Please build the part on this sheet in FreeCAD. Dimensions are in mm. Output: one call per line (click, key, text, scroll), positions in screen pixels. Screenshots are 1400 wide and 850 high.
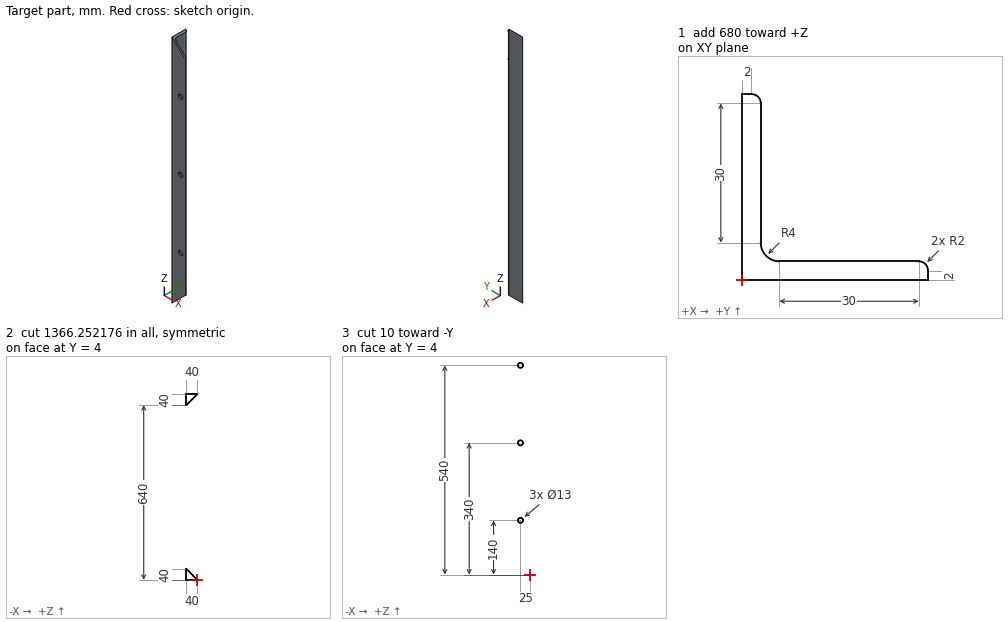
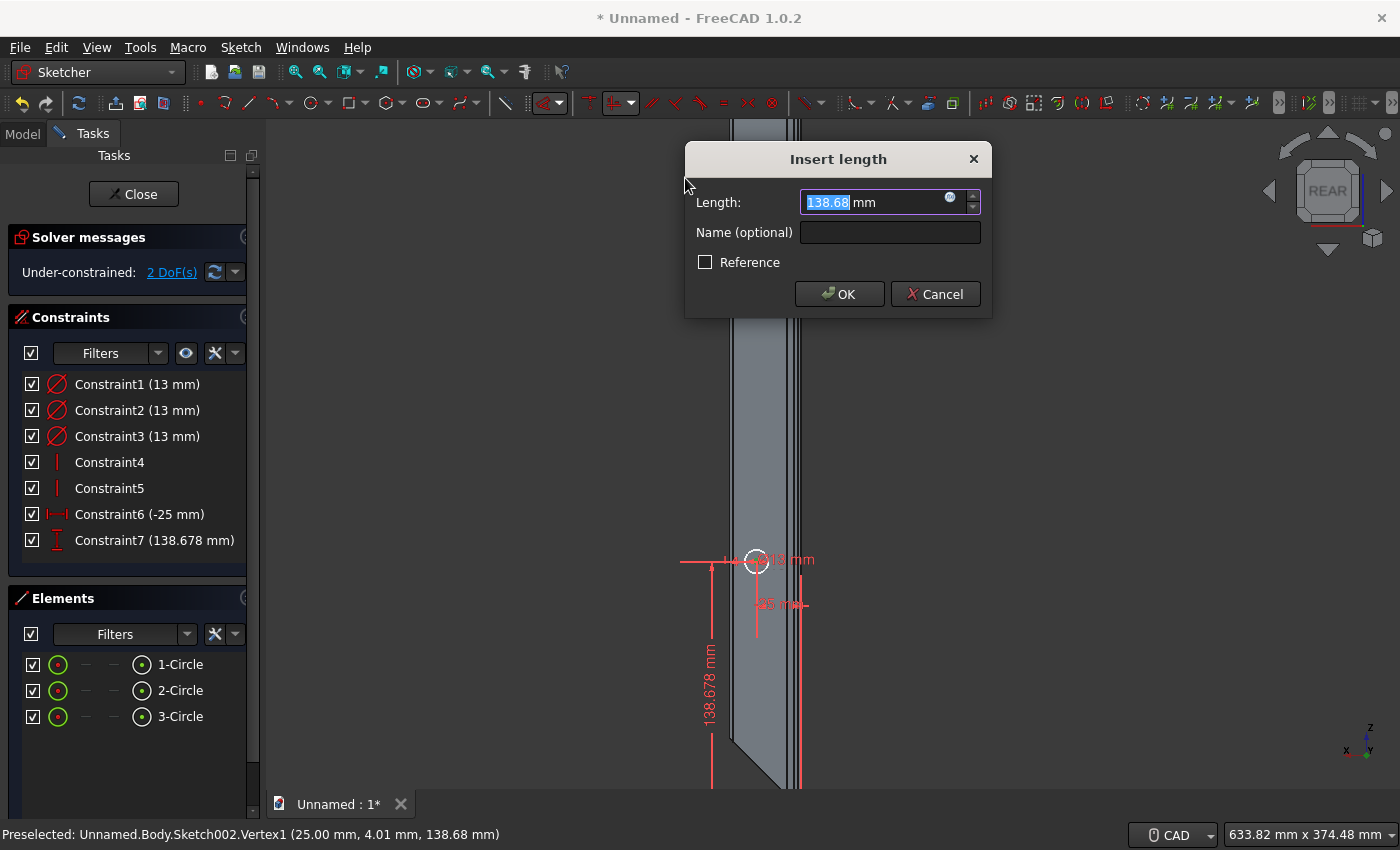
text(140)
key(Return)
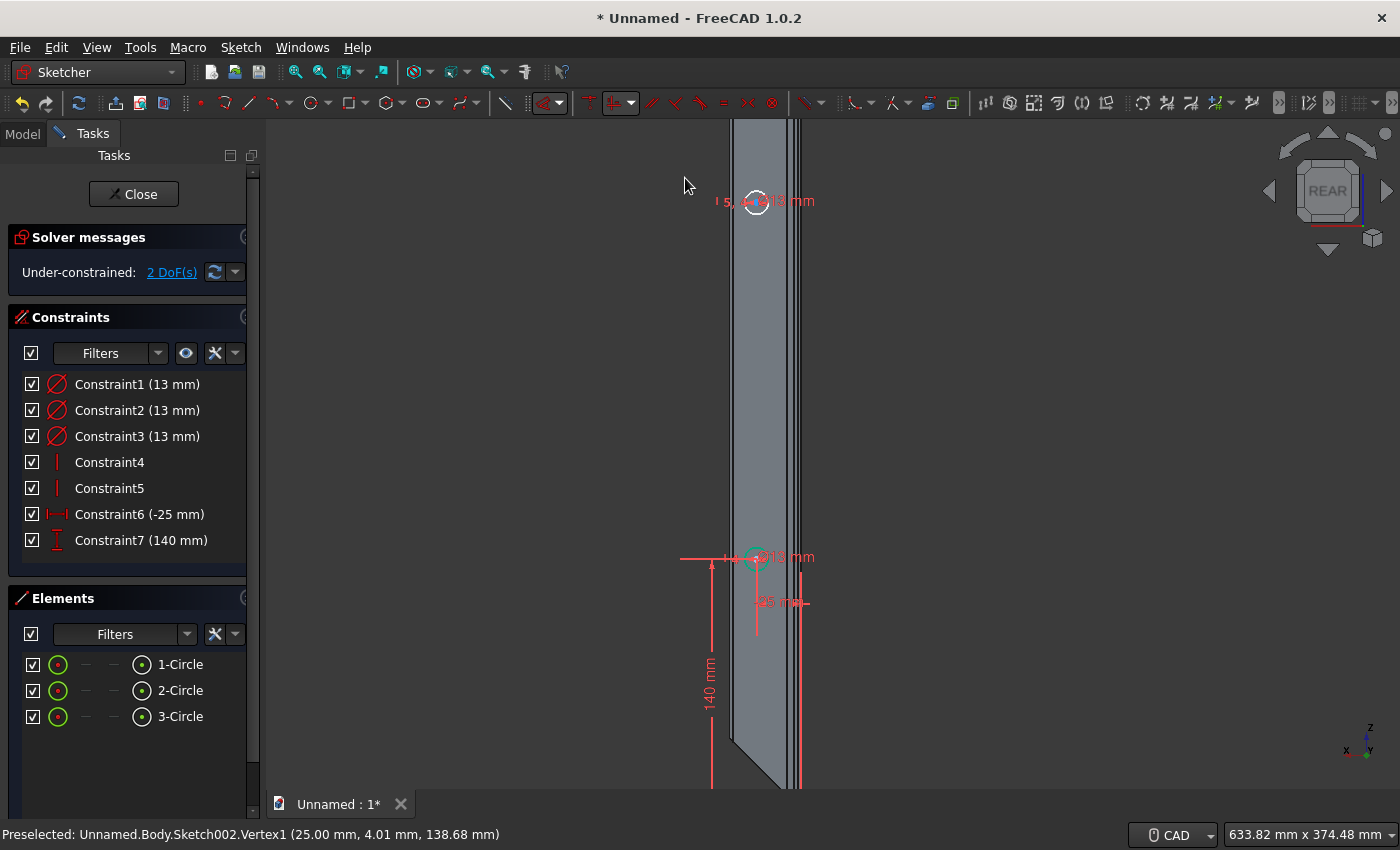
click(757, 203)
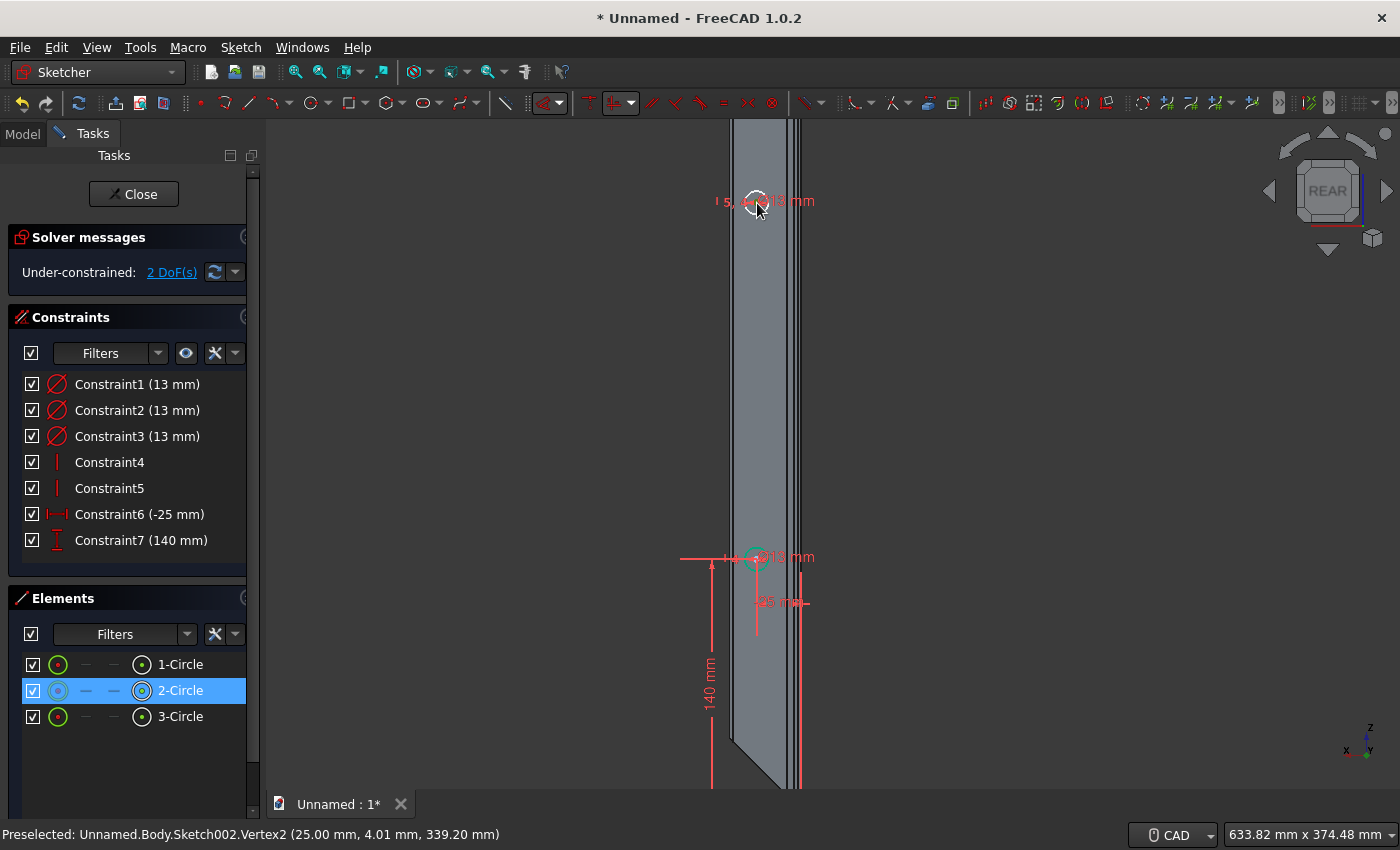
click(562, 104)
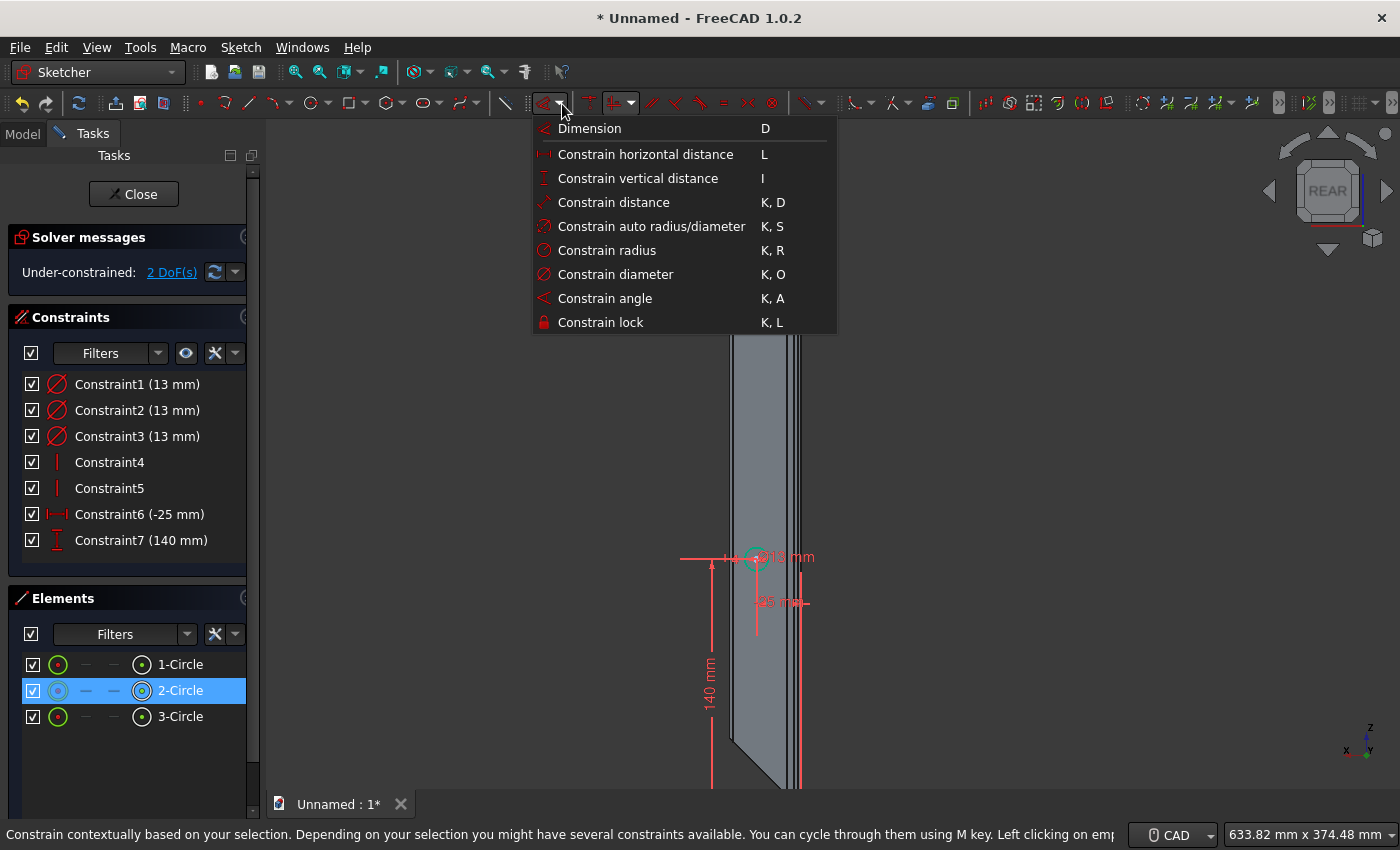
click(685, 178)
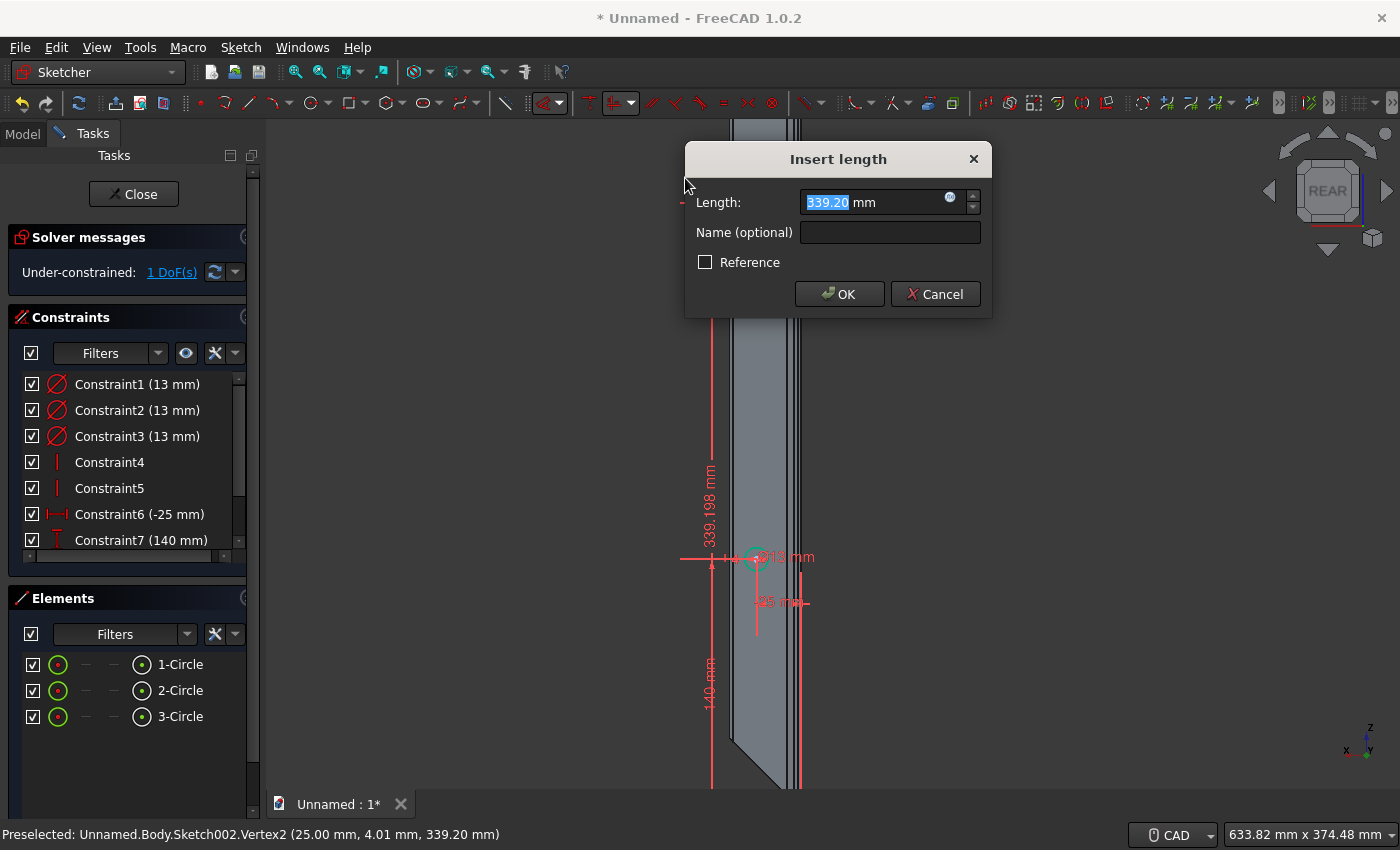
text(340)
key(Return)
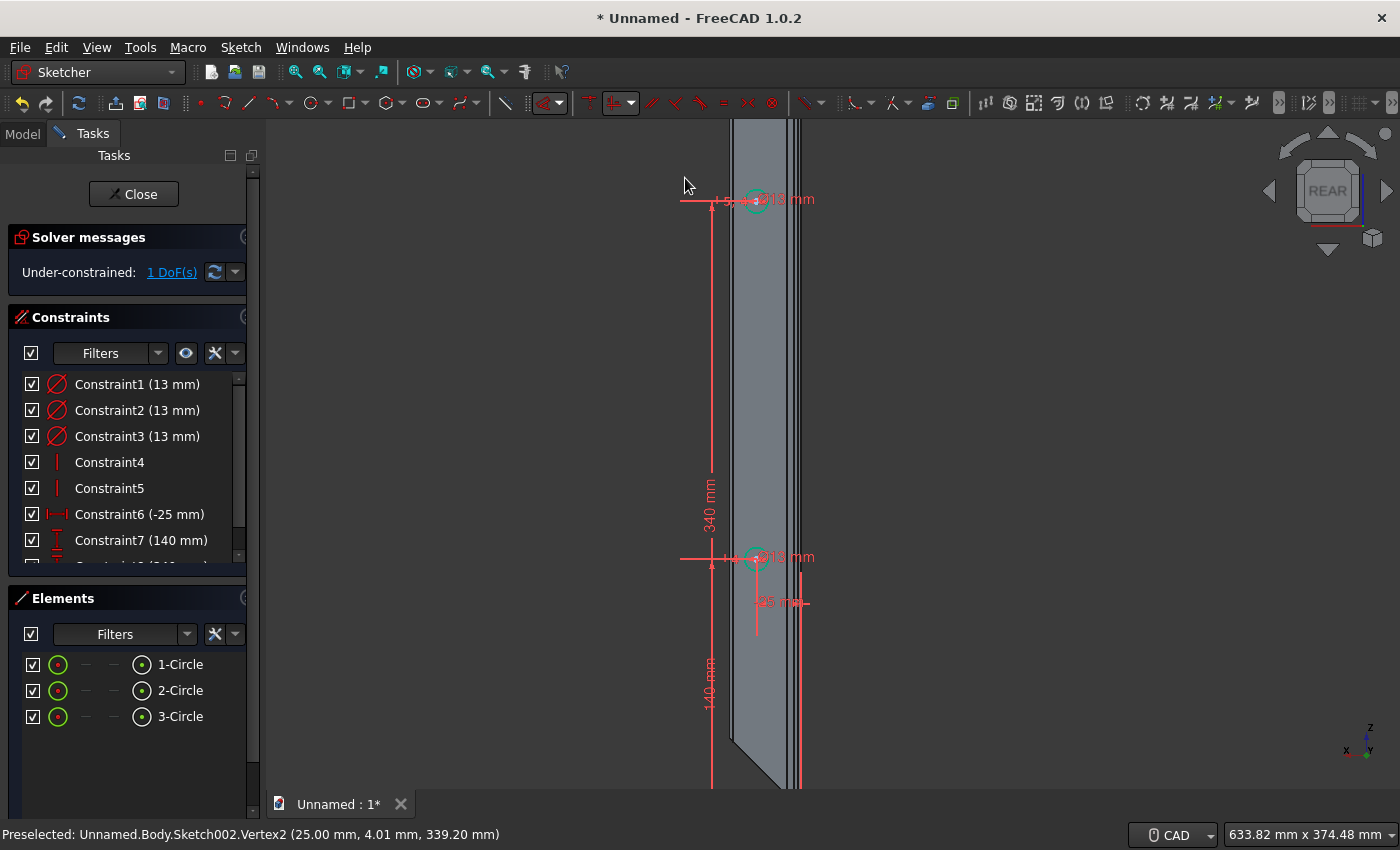
scroll(757, 563, down, 4)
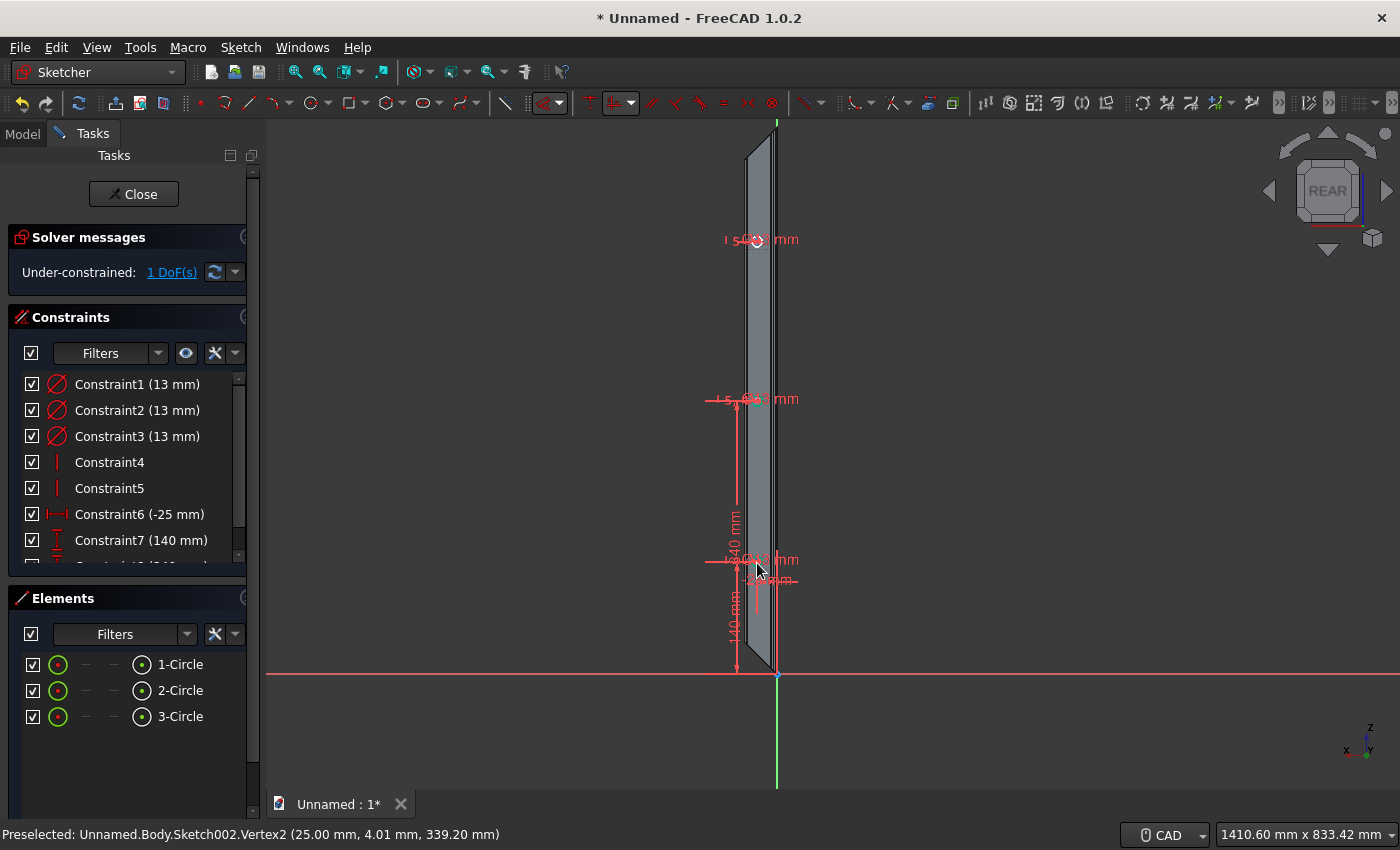
click(757, 242)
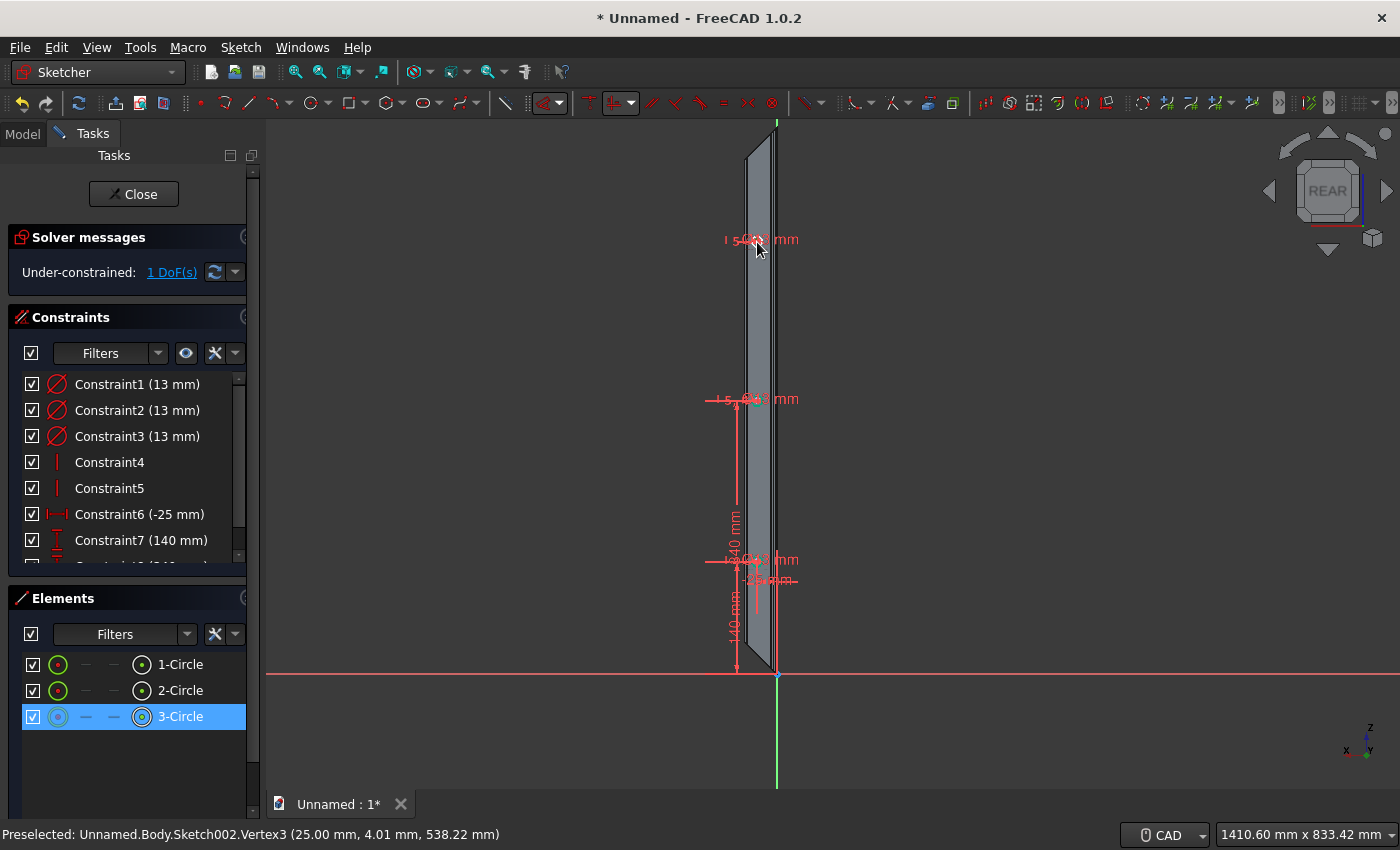
click(562, 104)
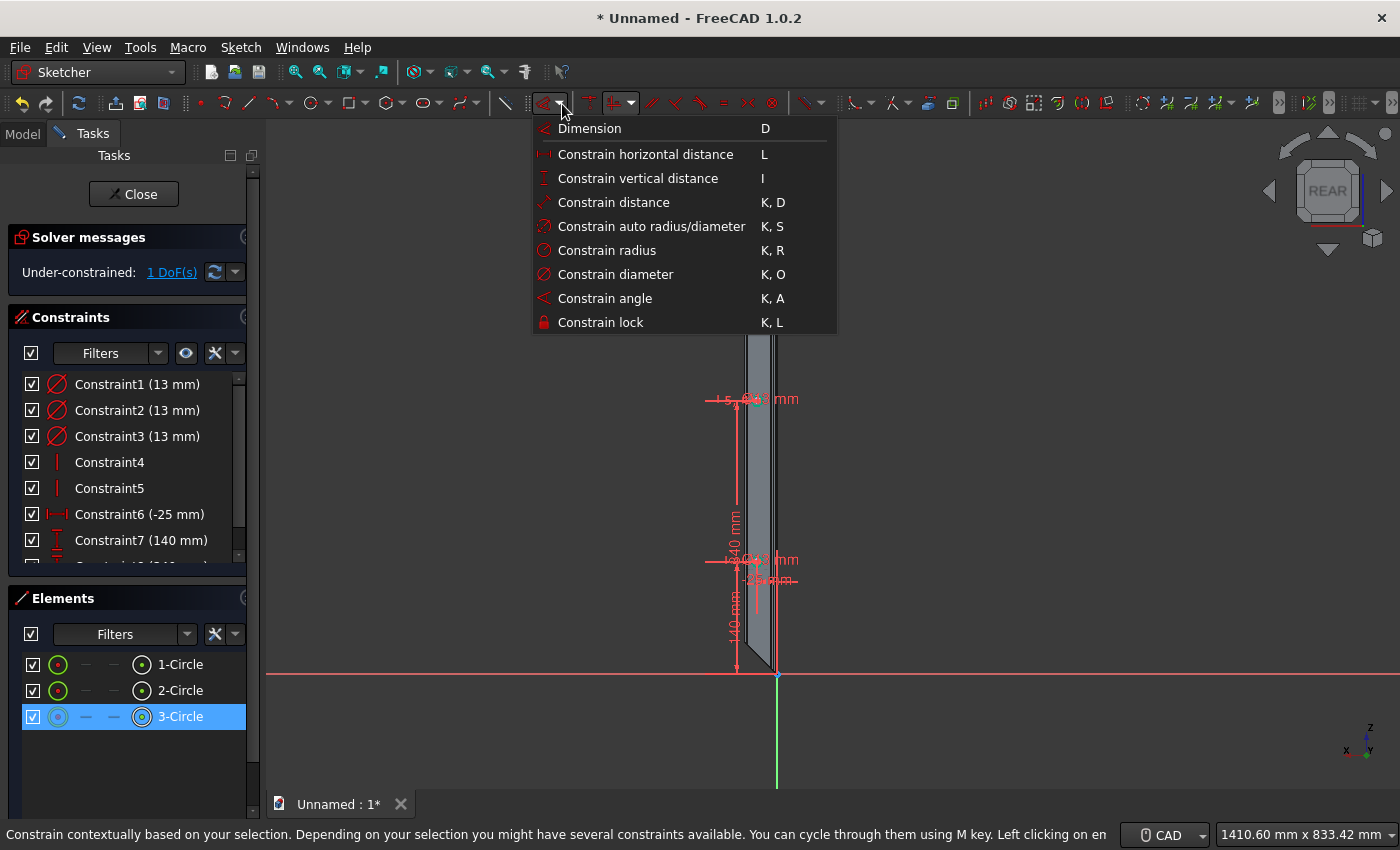
click(685, 178)